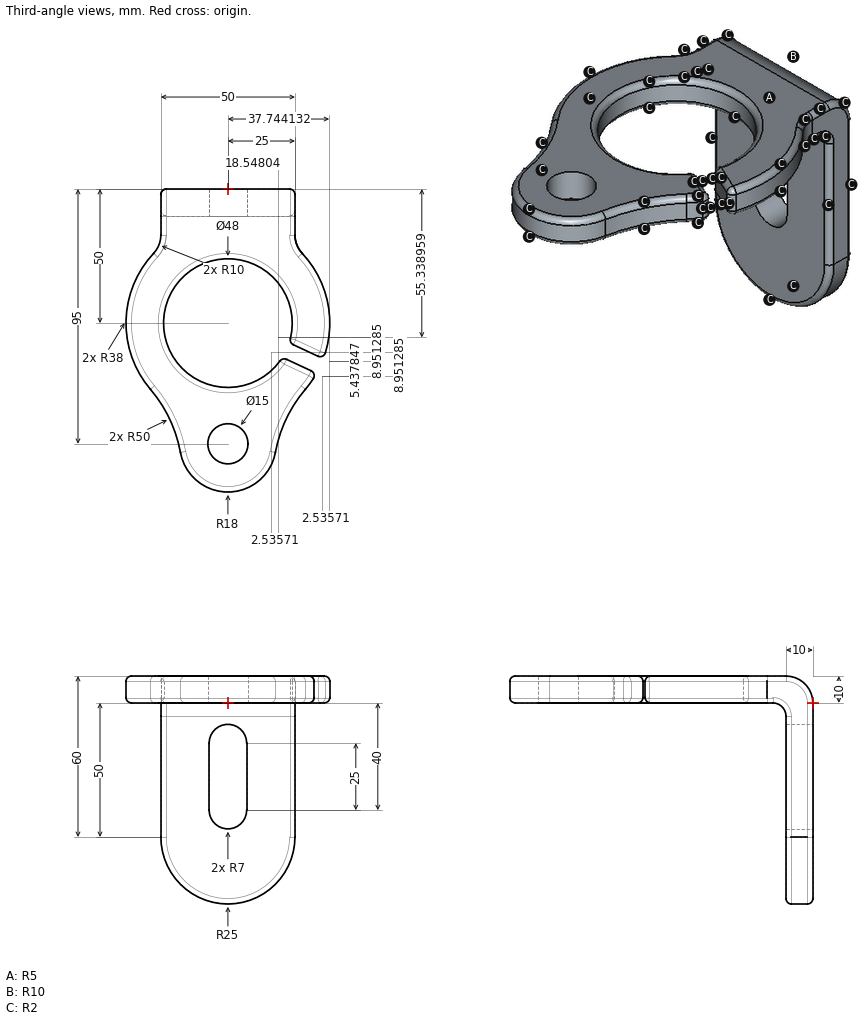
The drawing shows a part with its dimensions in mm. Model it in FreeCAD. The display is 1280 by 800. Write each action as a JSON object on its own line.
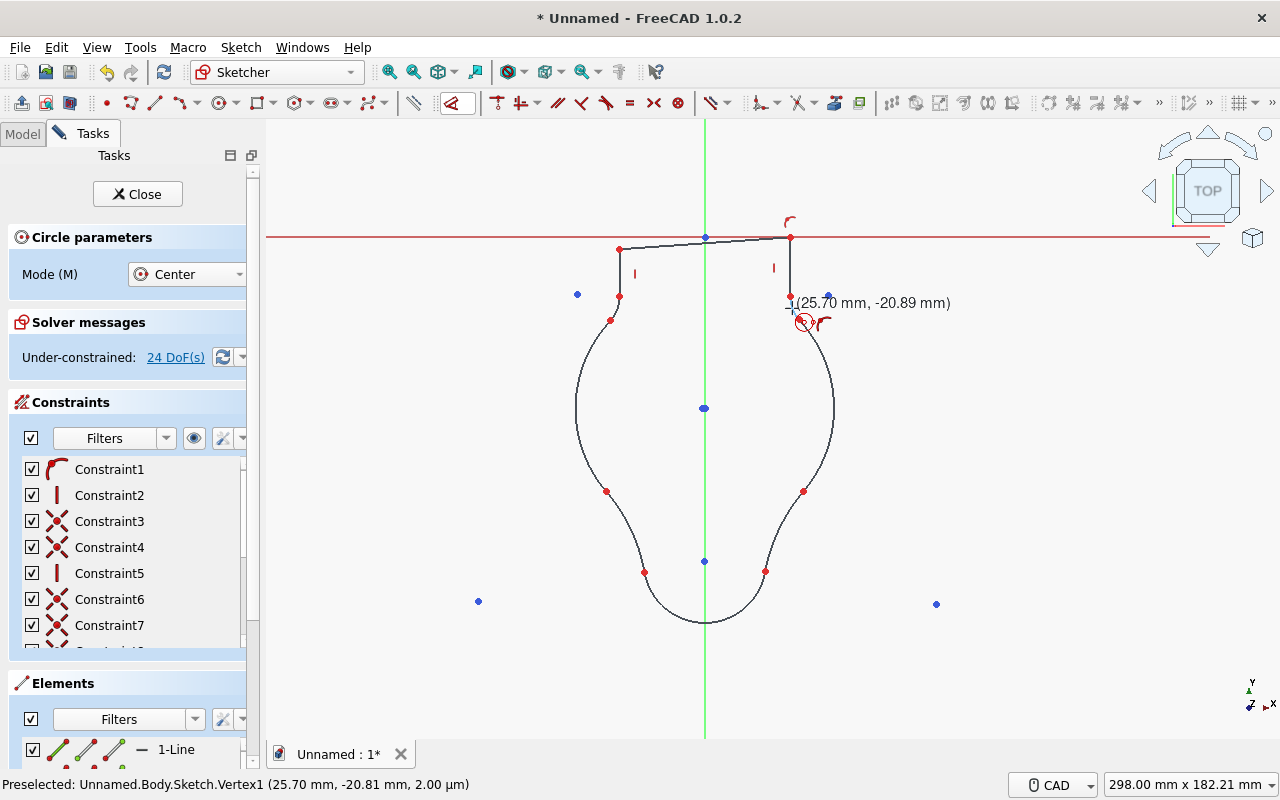
{"action": "left_click", "coordinate": [705, 561]}
{"action": "left_click", "coordinate": [723, 543]}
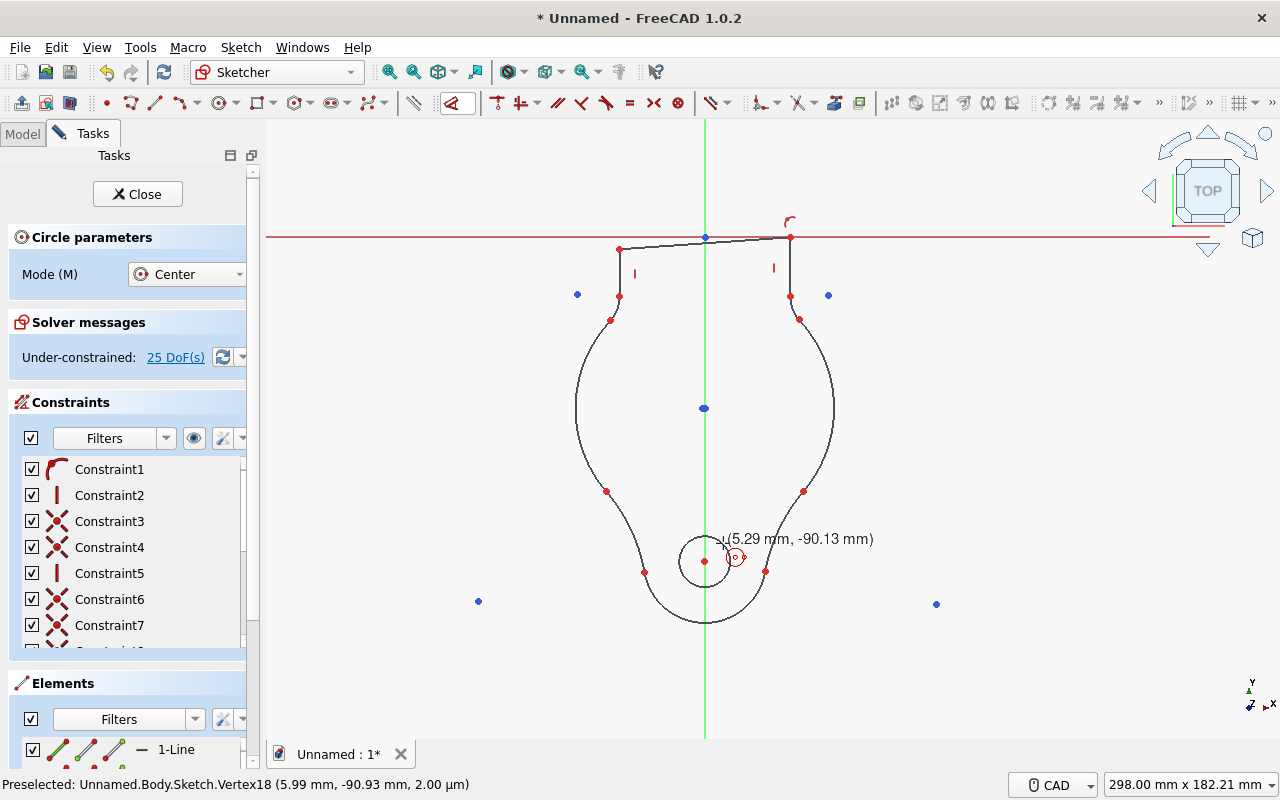
{"action": "left_click", "coordinate": [705, 407]}
{"action": "left_click", "coordinate": [763, 350]}
{"action": "key", "text": "Escape"}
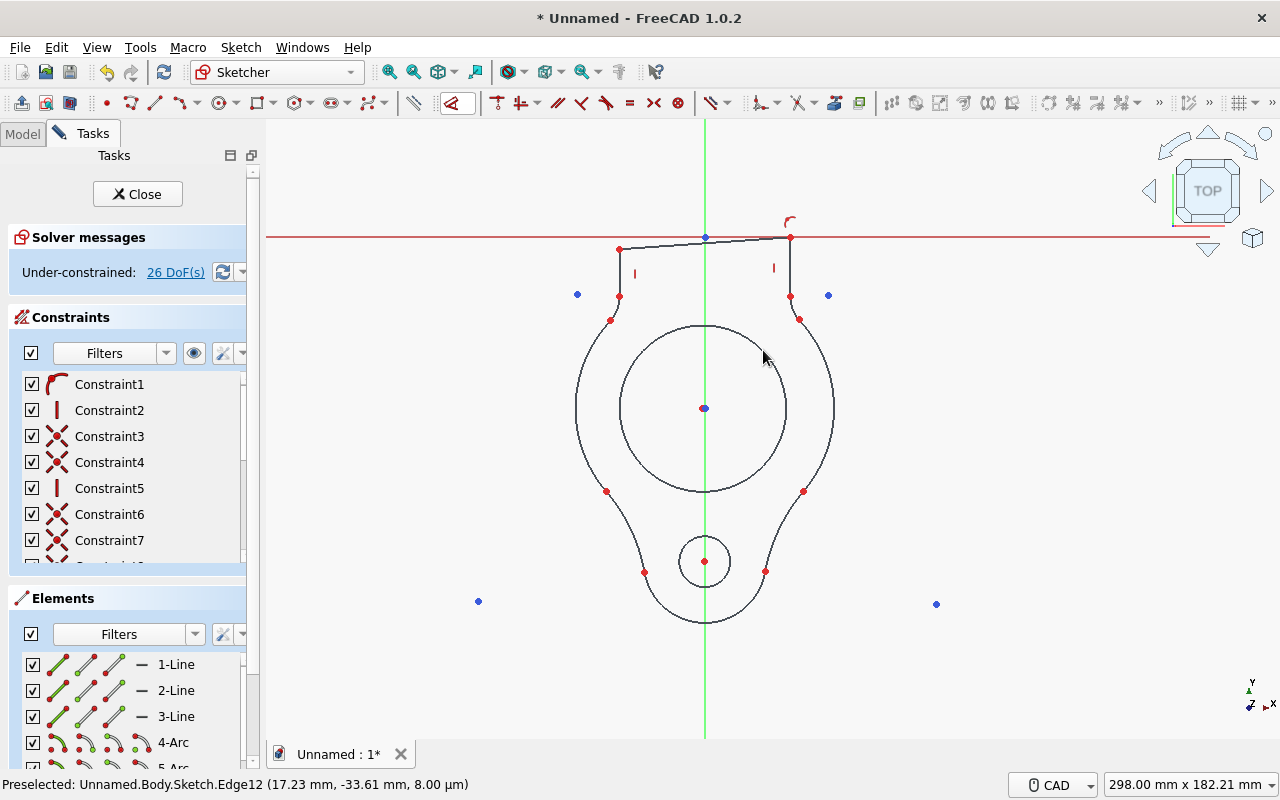
{"action": "left_click", "coordinate": [790, 279]}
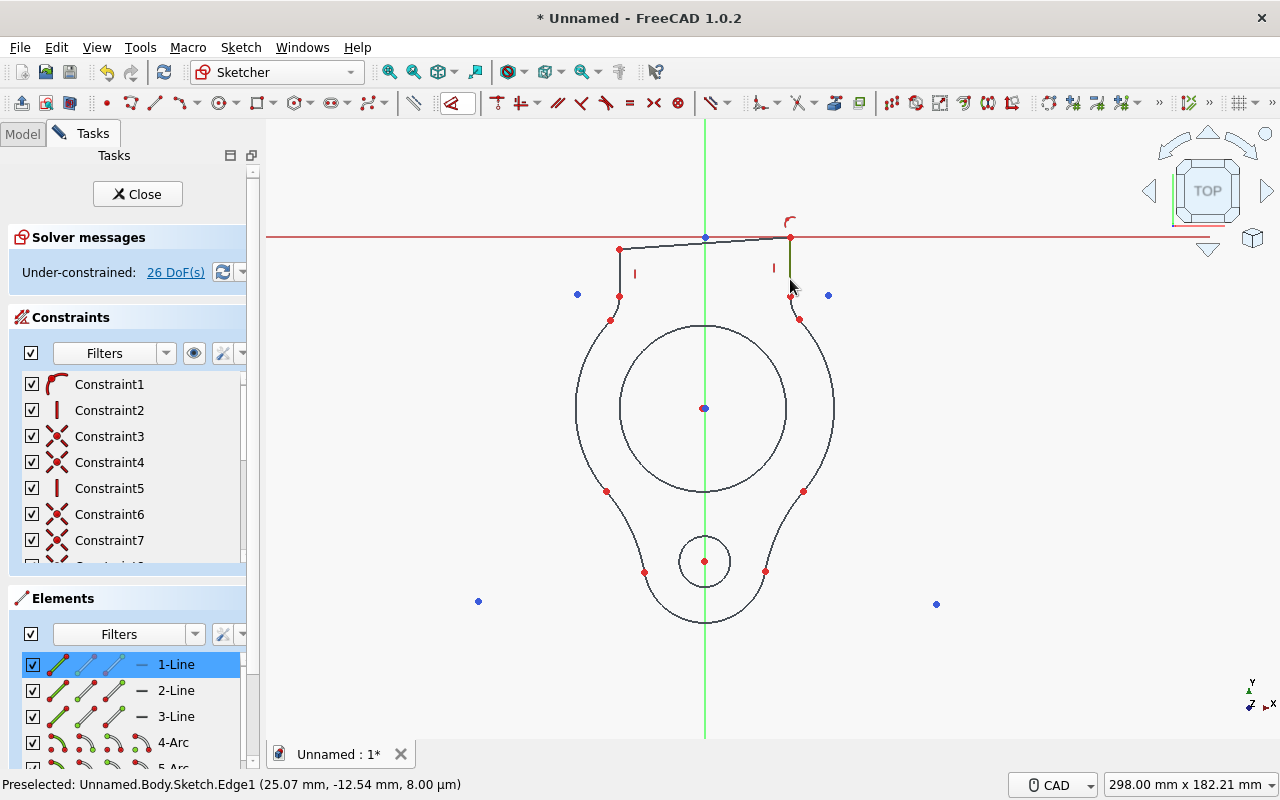
{"action": "left_click", "coordinate": [793, 309]}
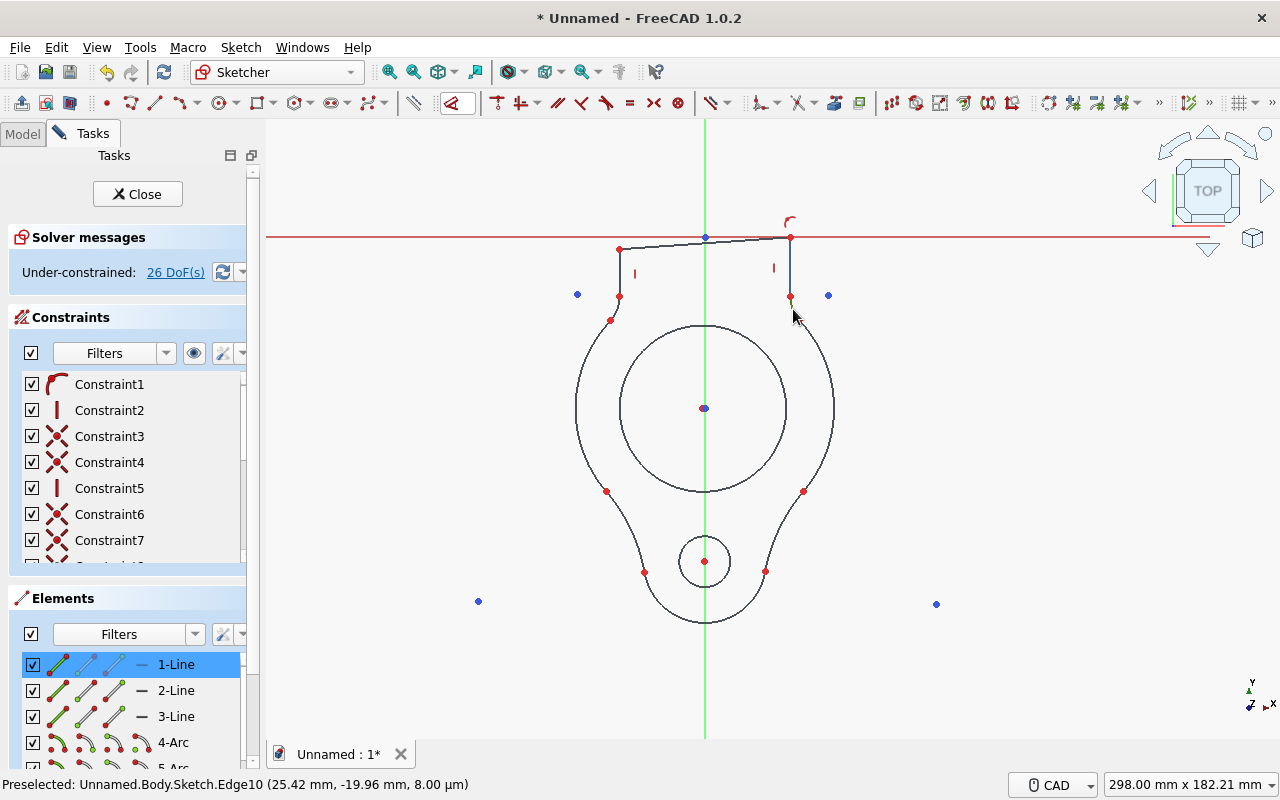
{"action": "left_click", "coordinate": [606, 104]}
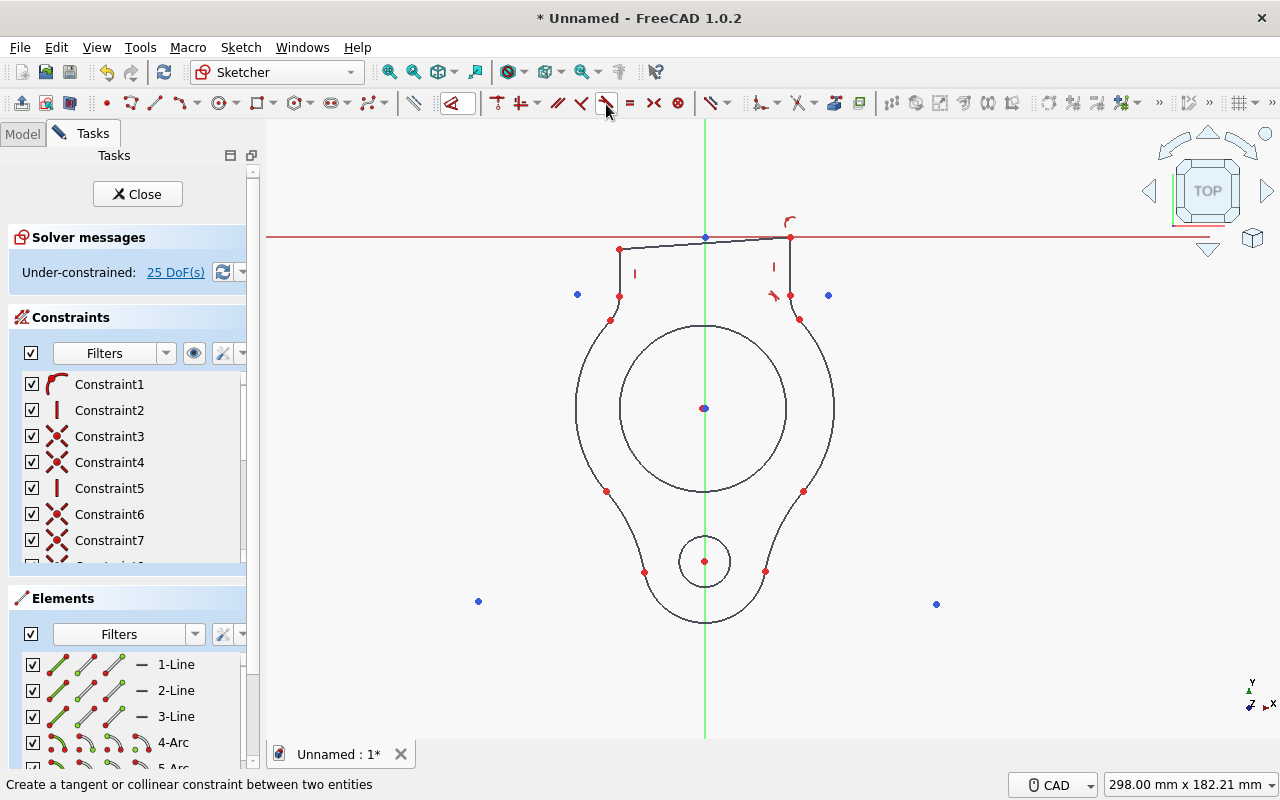
{"action": "left_click", "coordinate": [620, 264]}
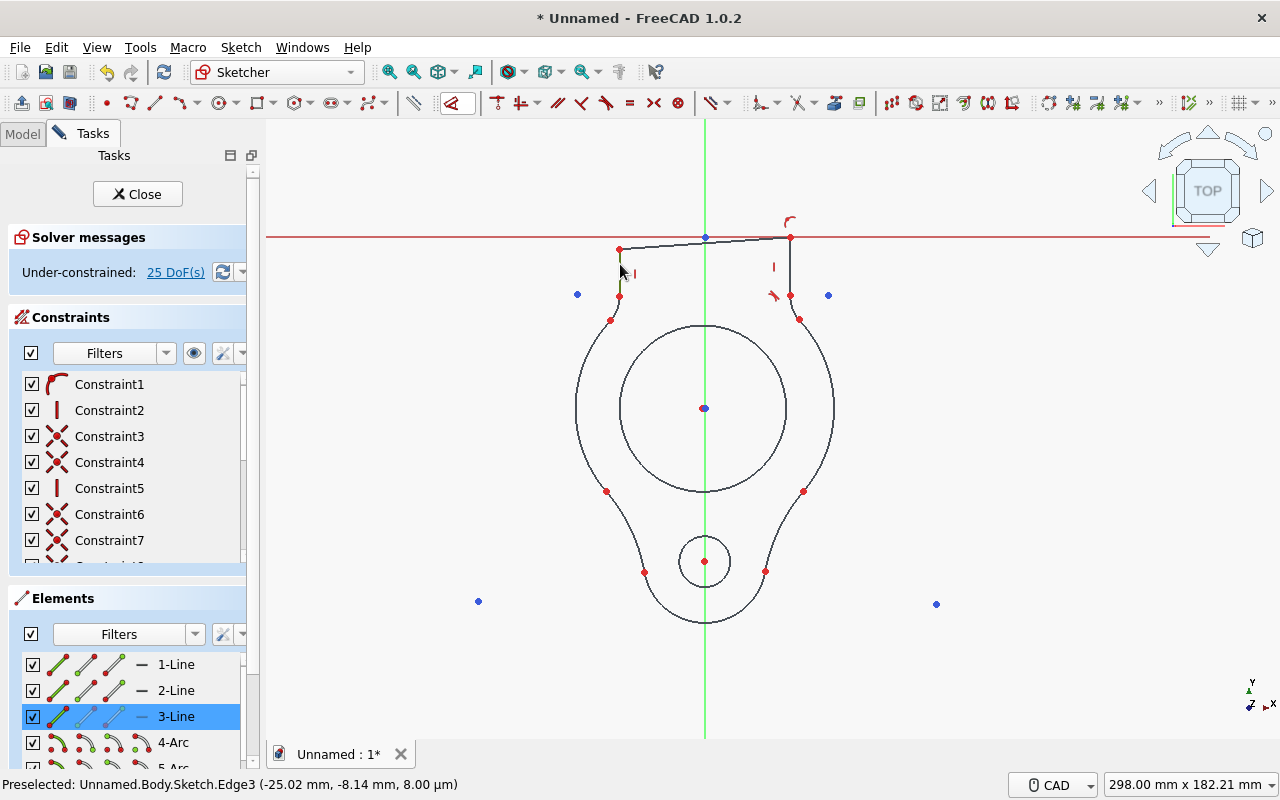
{"action": "left_click", "coordinate": [617, 309]}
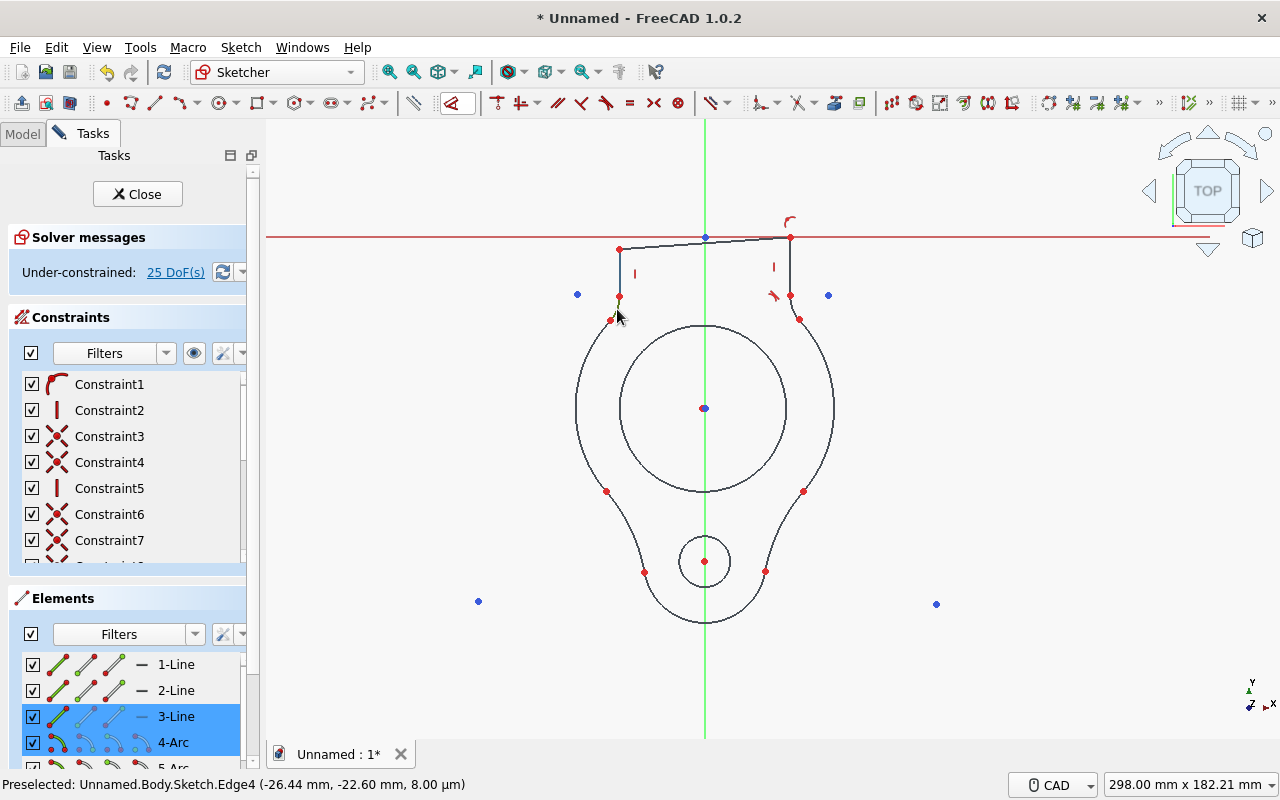
{"action": "left_click", "coordinate": [606, 104]}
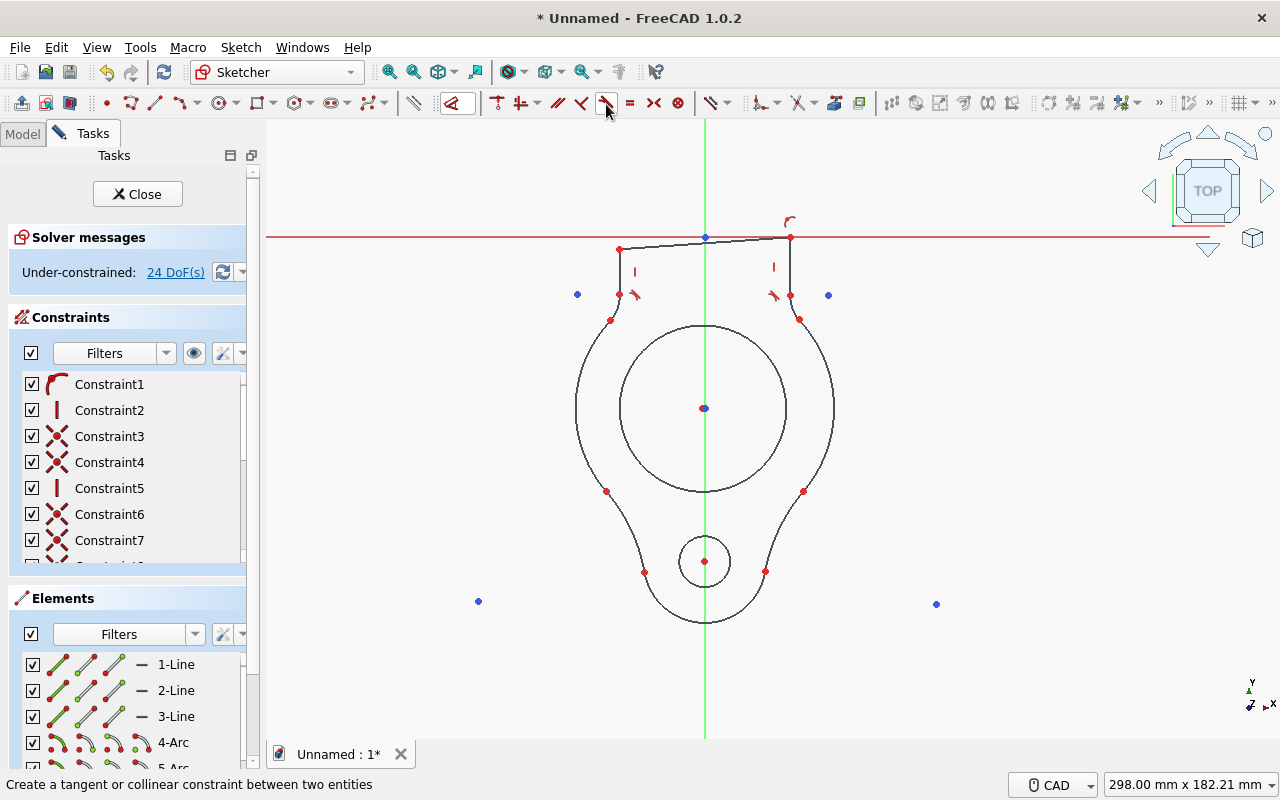
{"action": "left_click", "coordinate": [618, 308]}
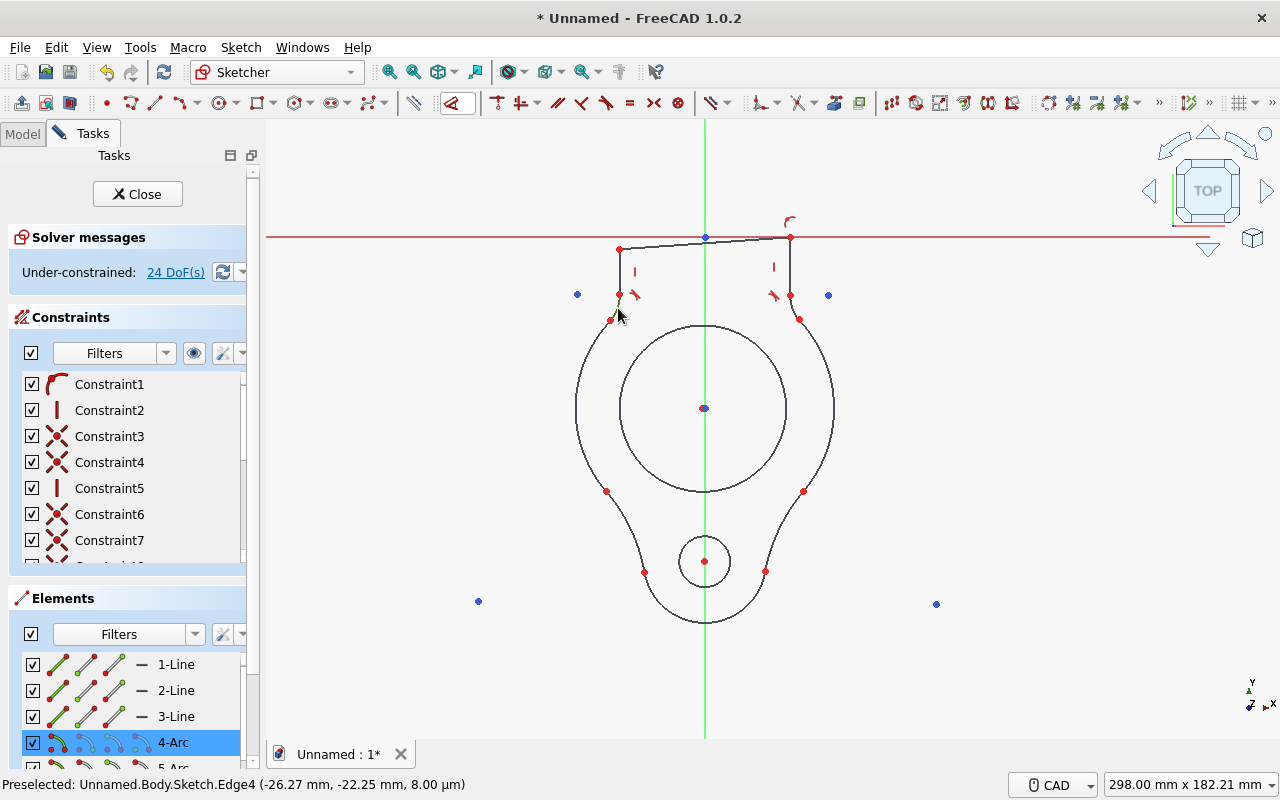
{"action": "left_click", "coordinate": [582, 369]}